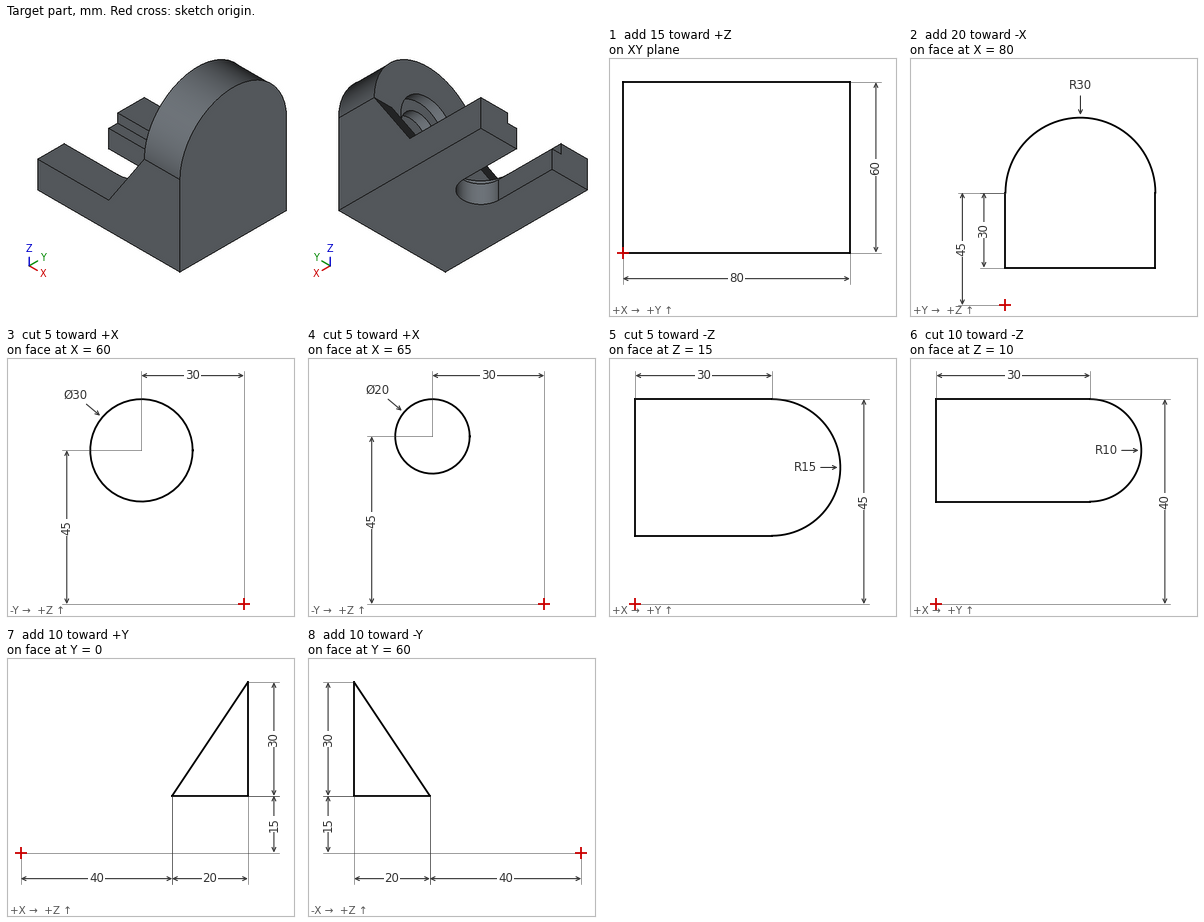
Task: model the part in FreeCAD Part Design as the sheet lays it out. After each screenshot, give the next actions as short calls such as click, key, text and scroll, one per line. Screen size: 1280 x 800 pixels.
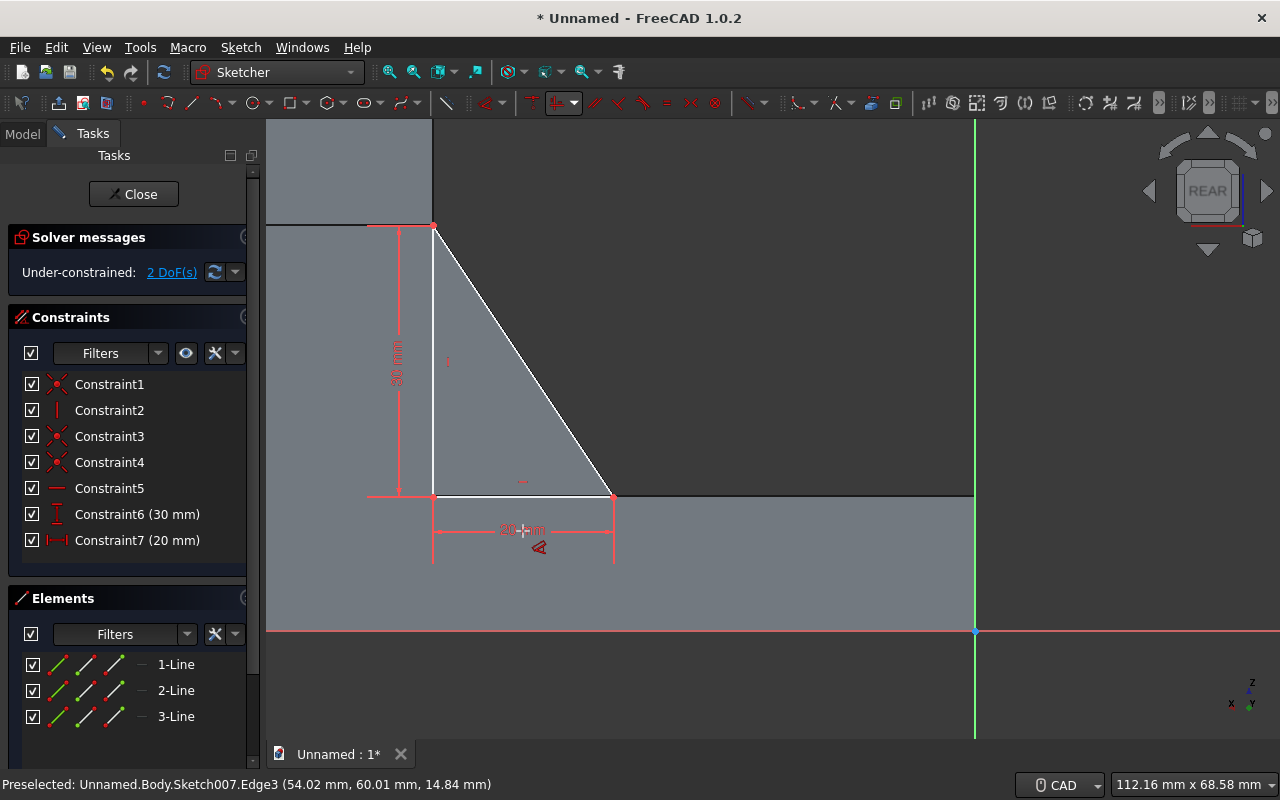
click(614, 497)
click(795, 665)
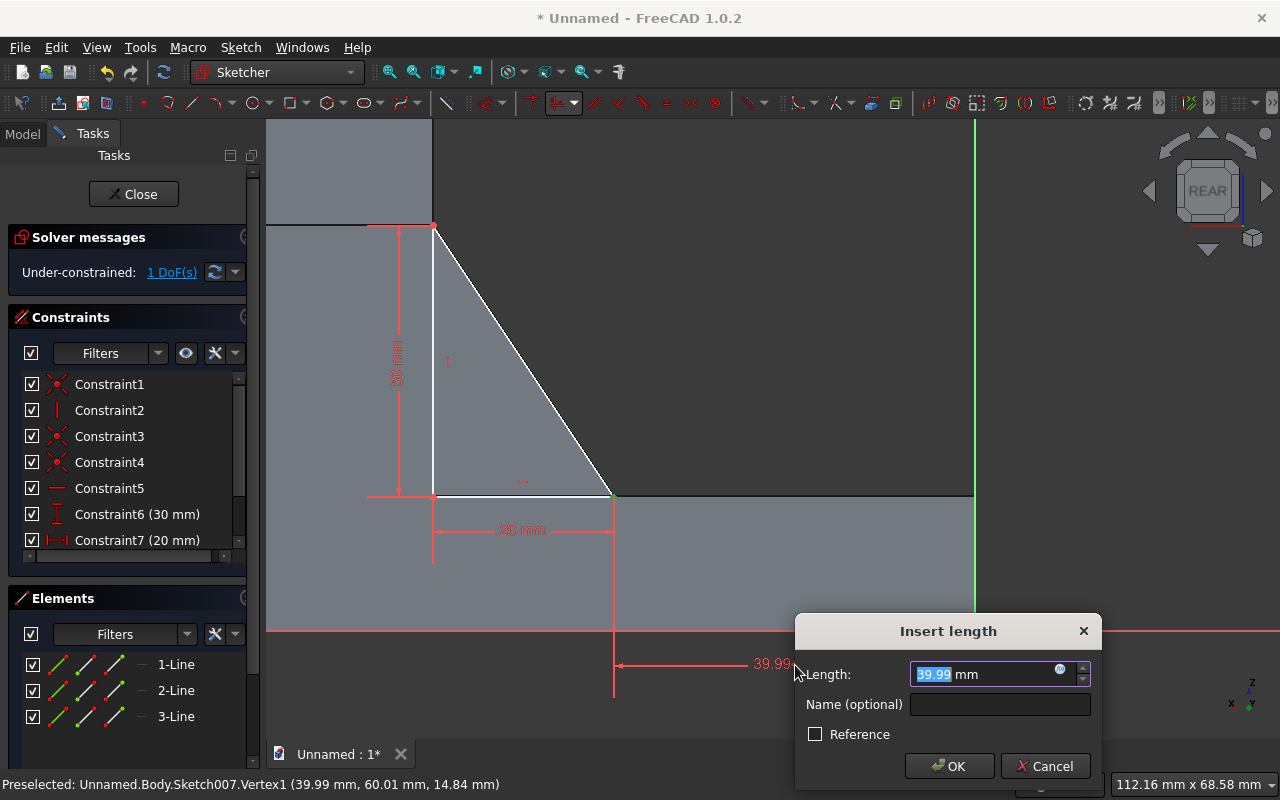
text(40)
key(Return)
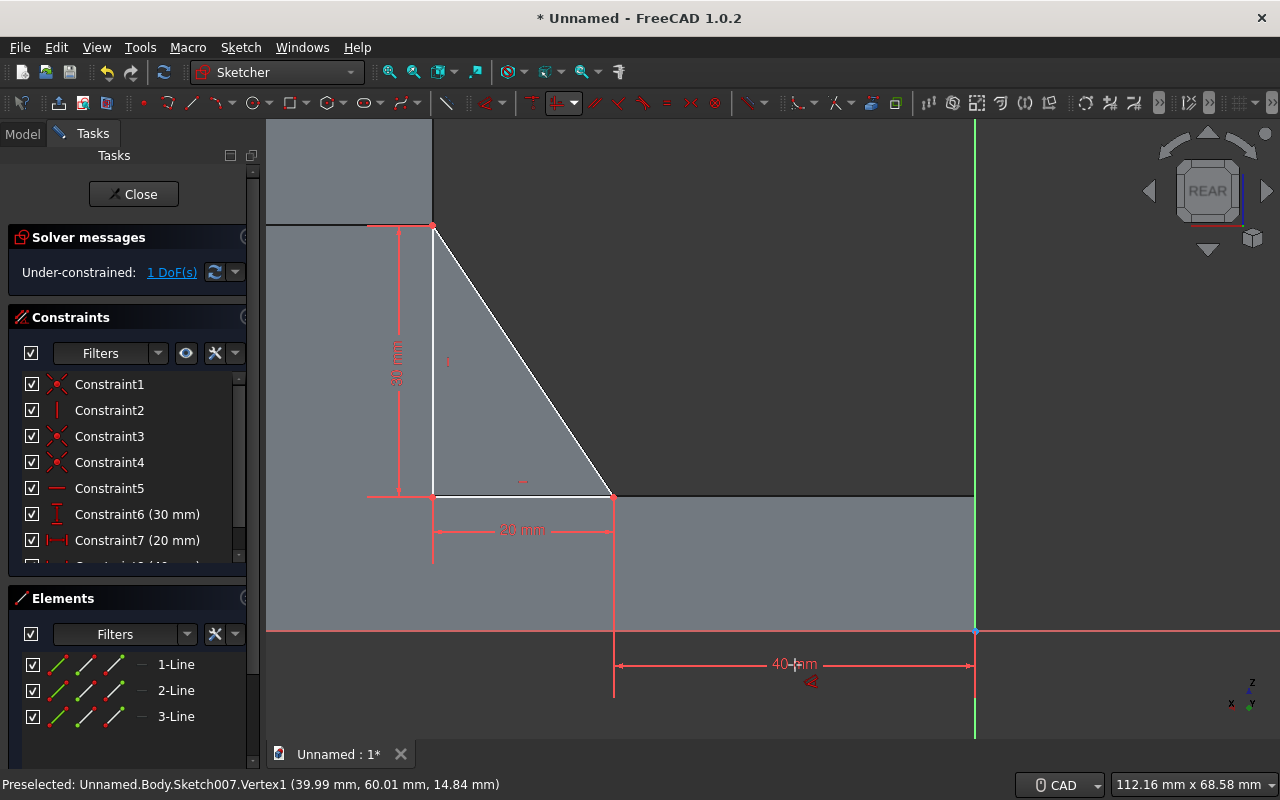
click(614, 497)
click(1009, 564)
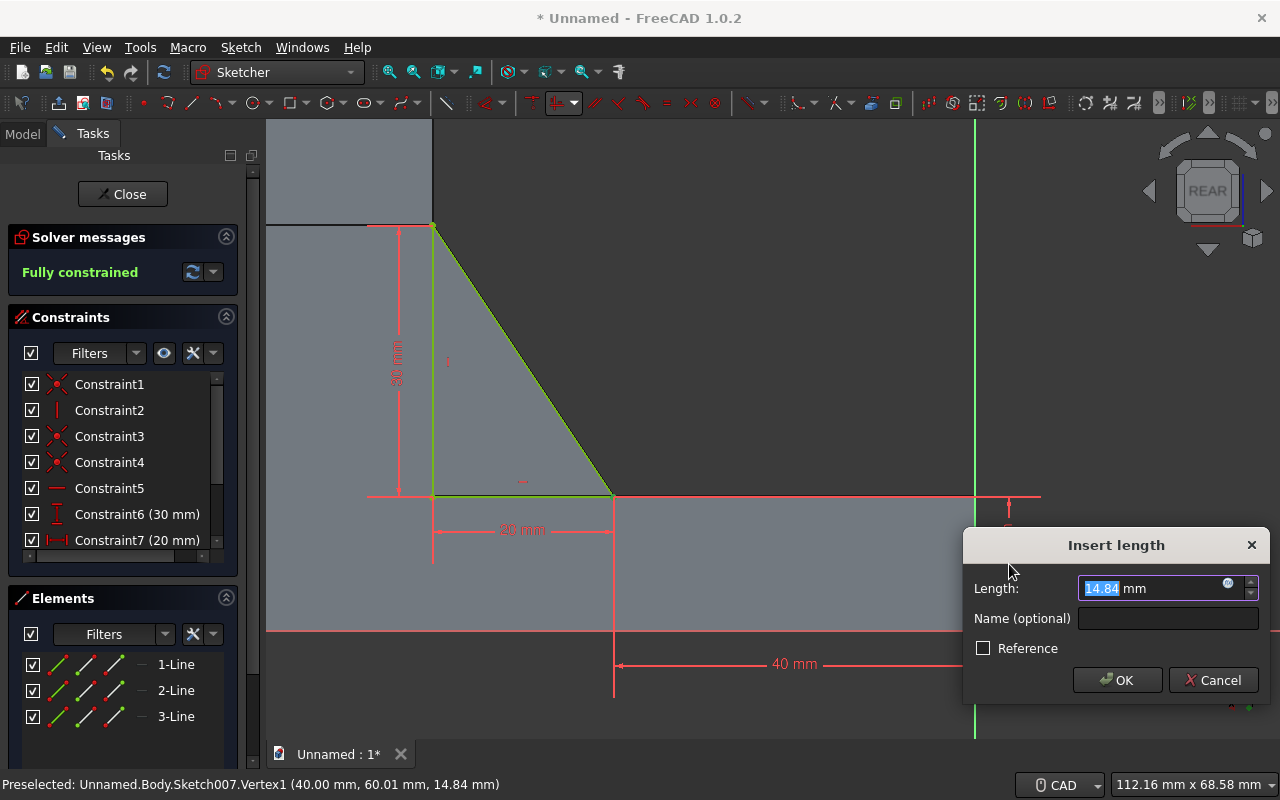
text(15)
key(Return)
key(Escape)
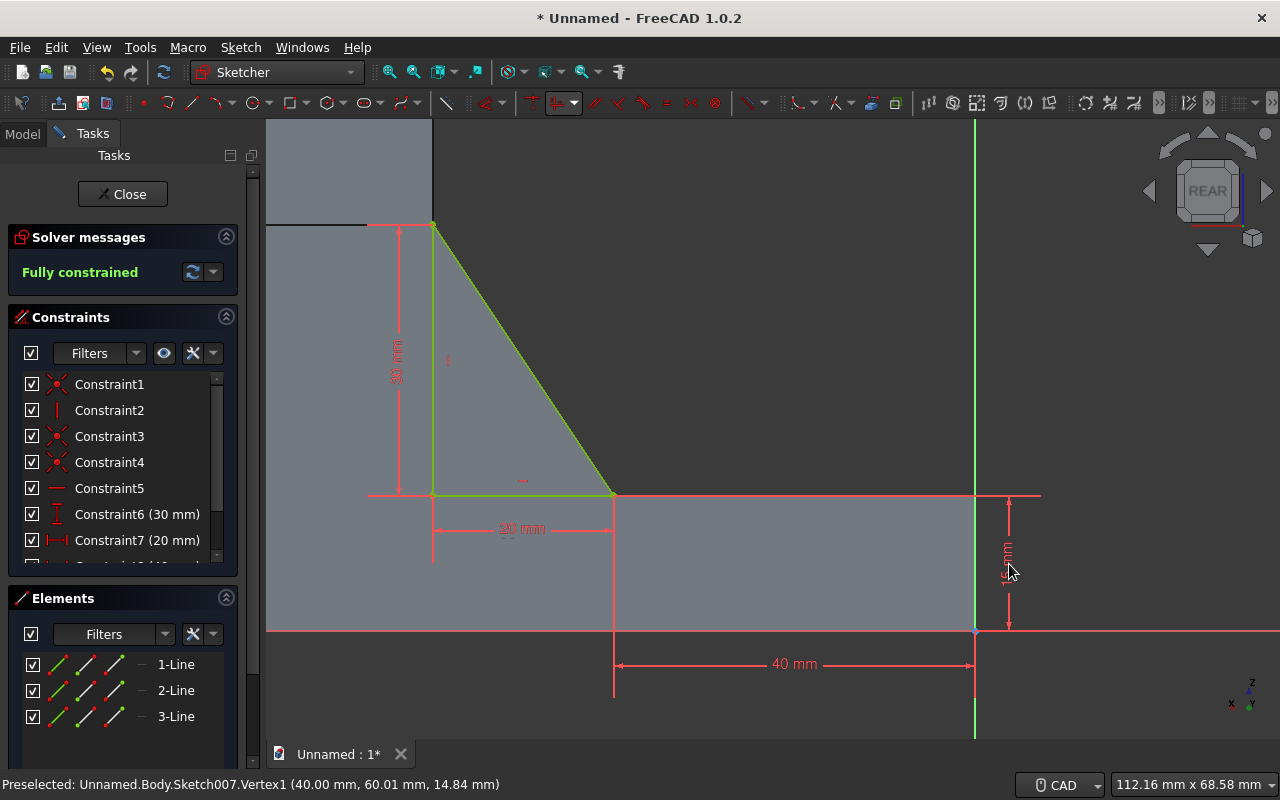
click(123, 194)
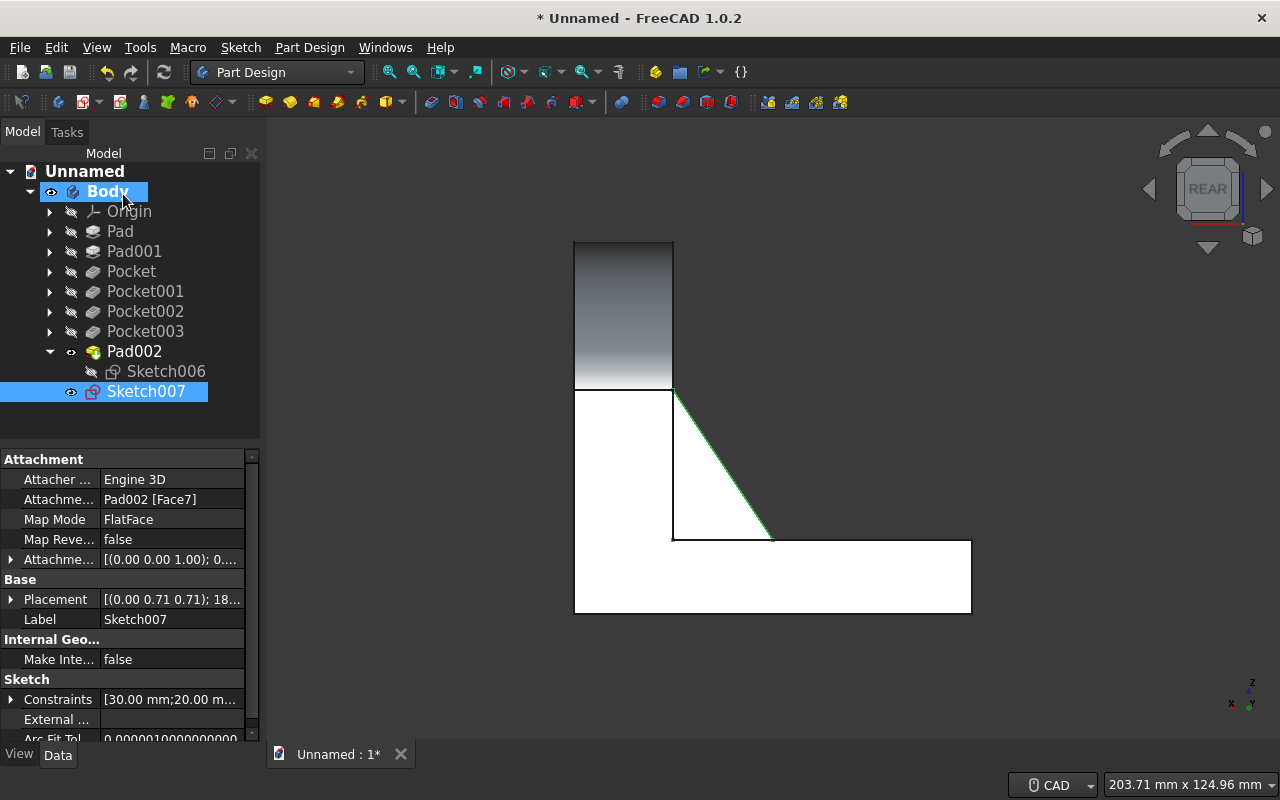
click(266, 102)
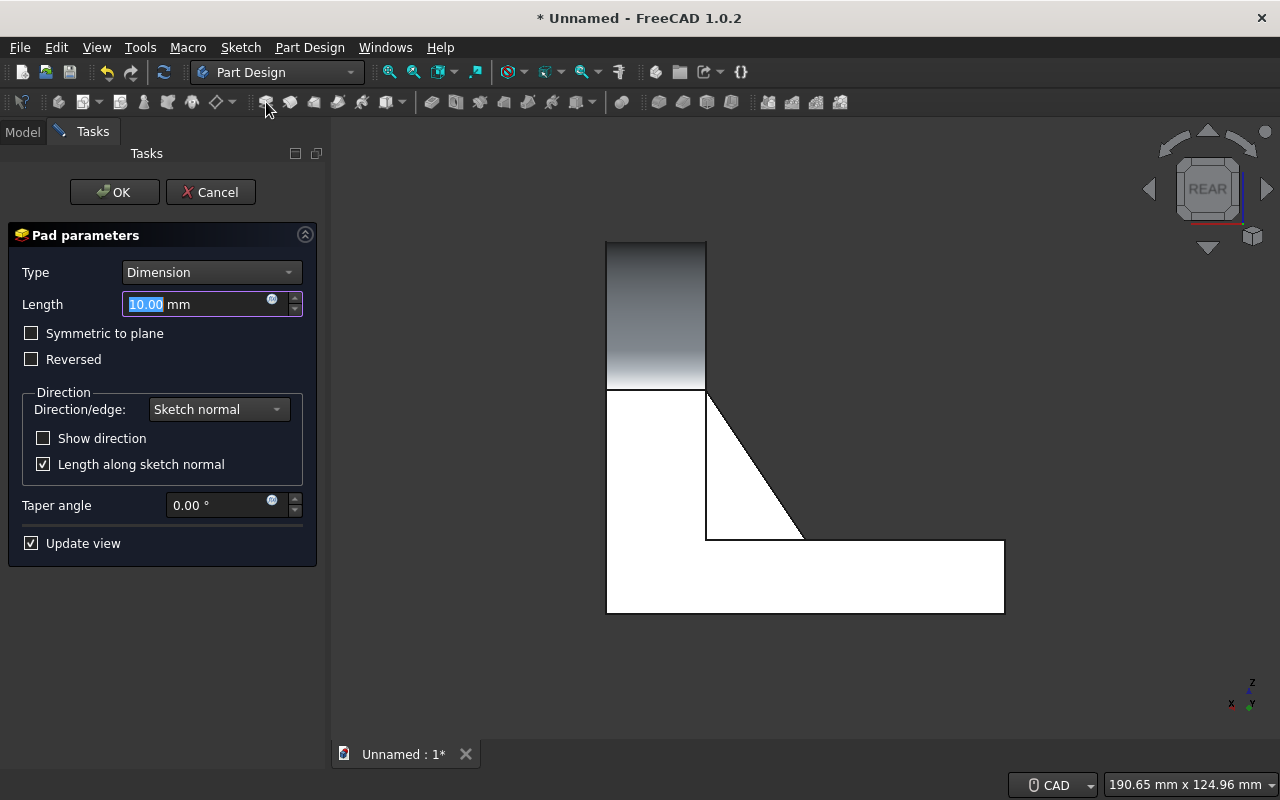
text(10)
key(Tab)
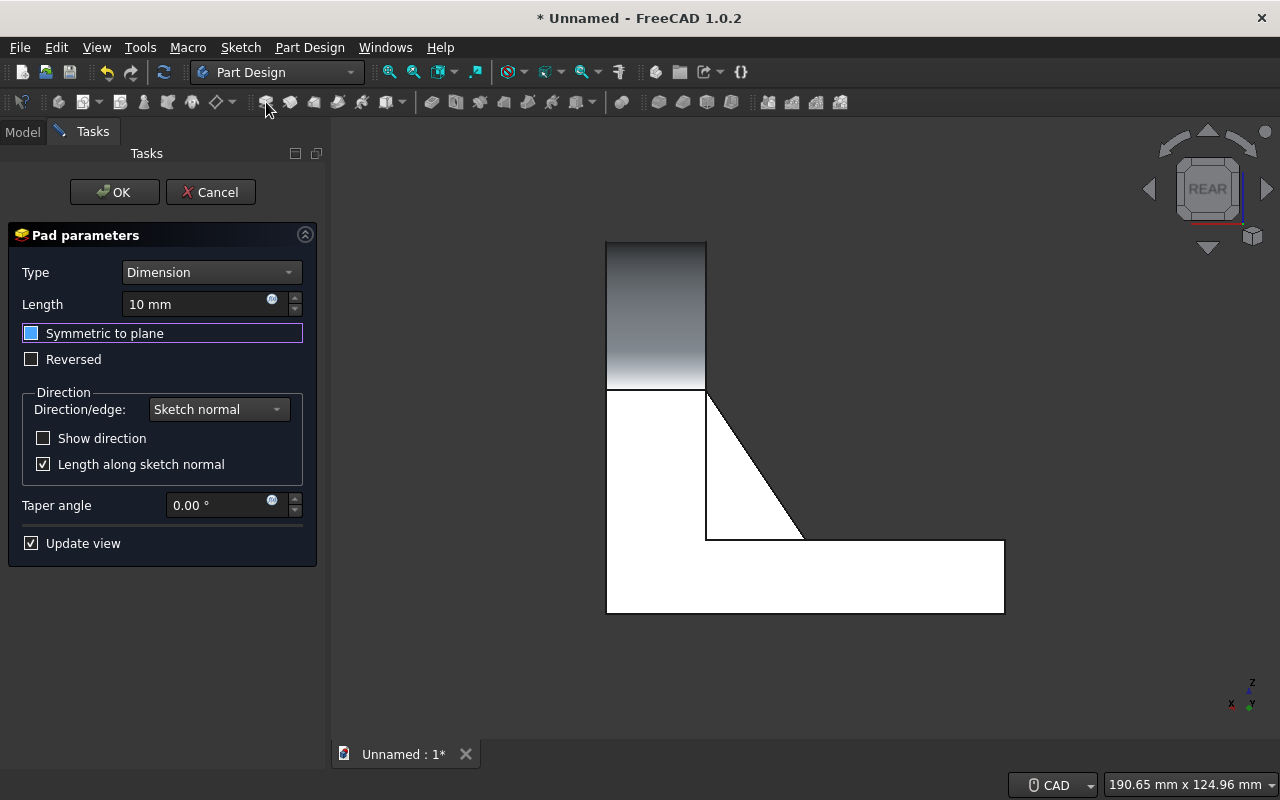
click(30, 359)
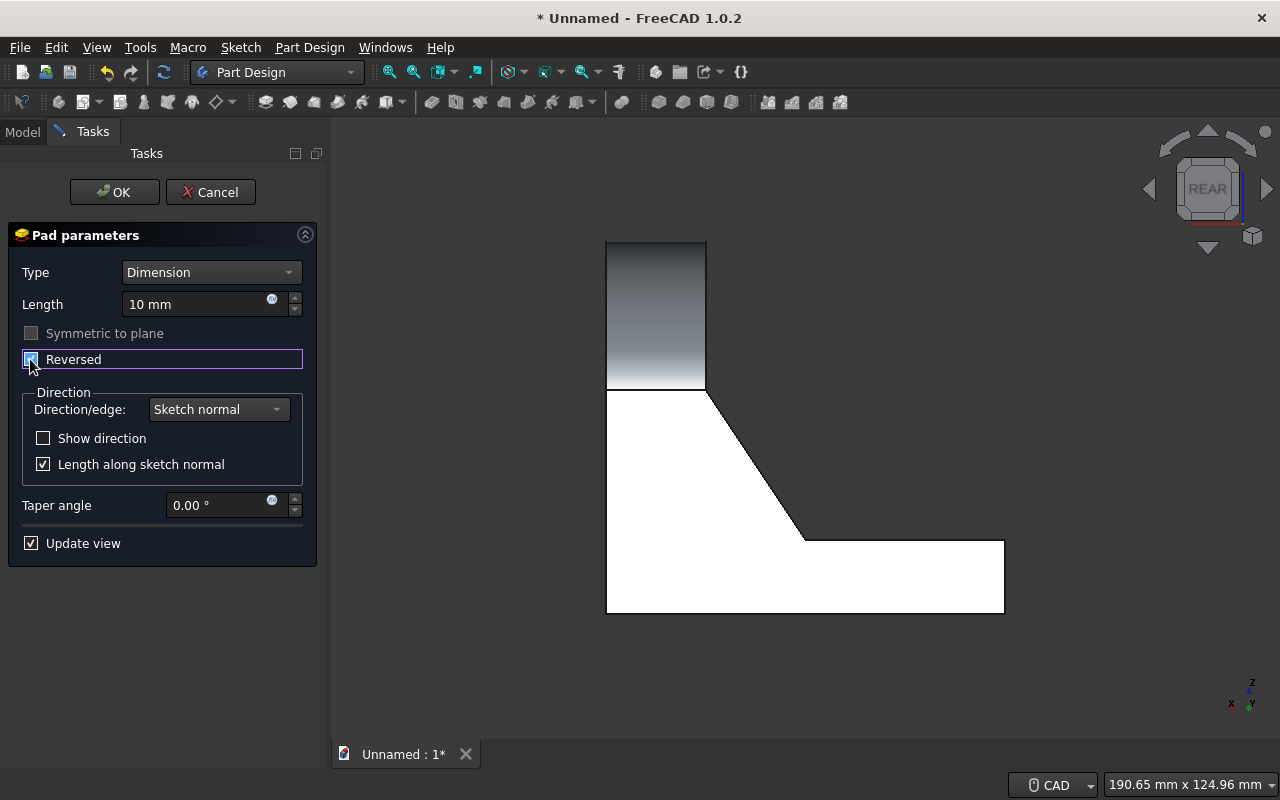
click(115, 192)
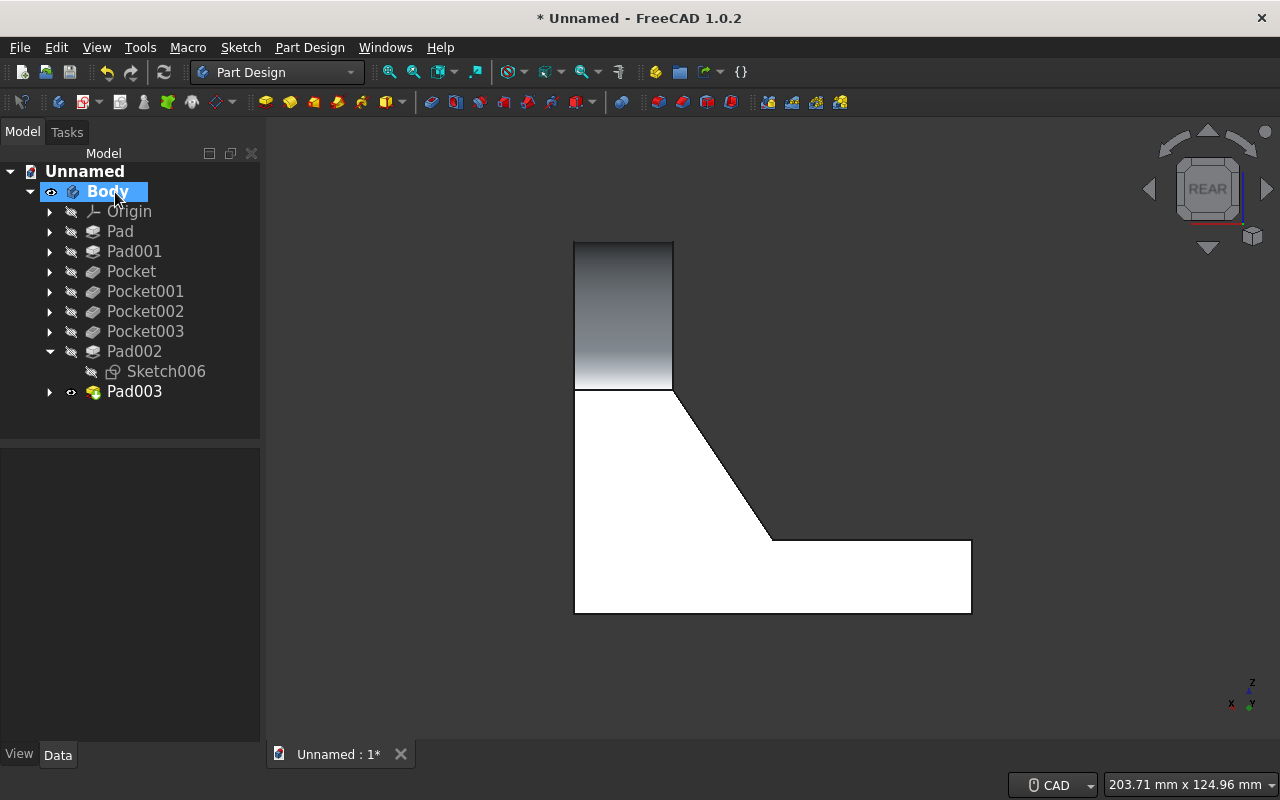
key(0)